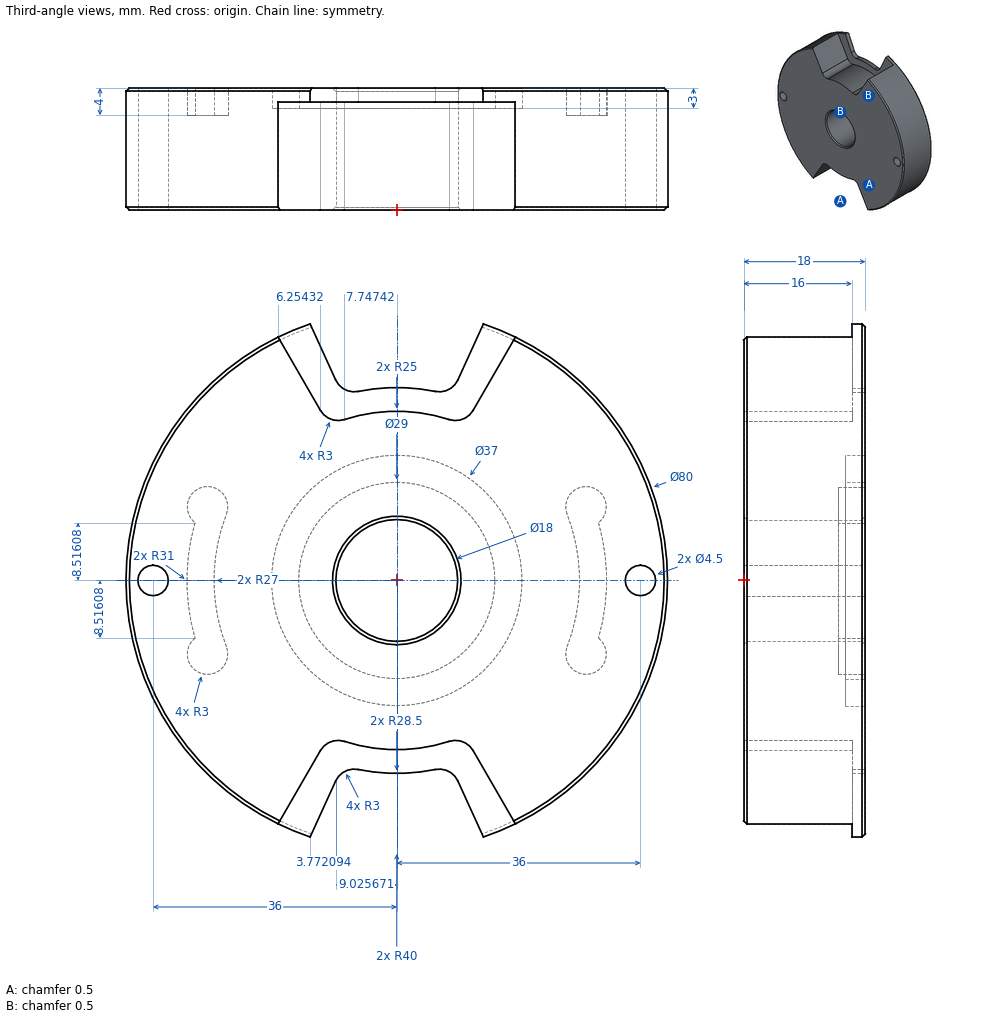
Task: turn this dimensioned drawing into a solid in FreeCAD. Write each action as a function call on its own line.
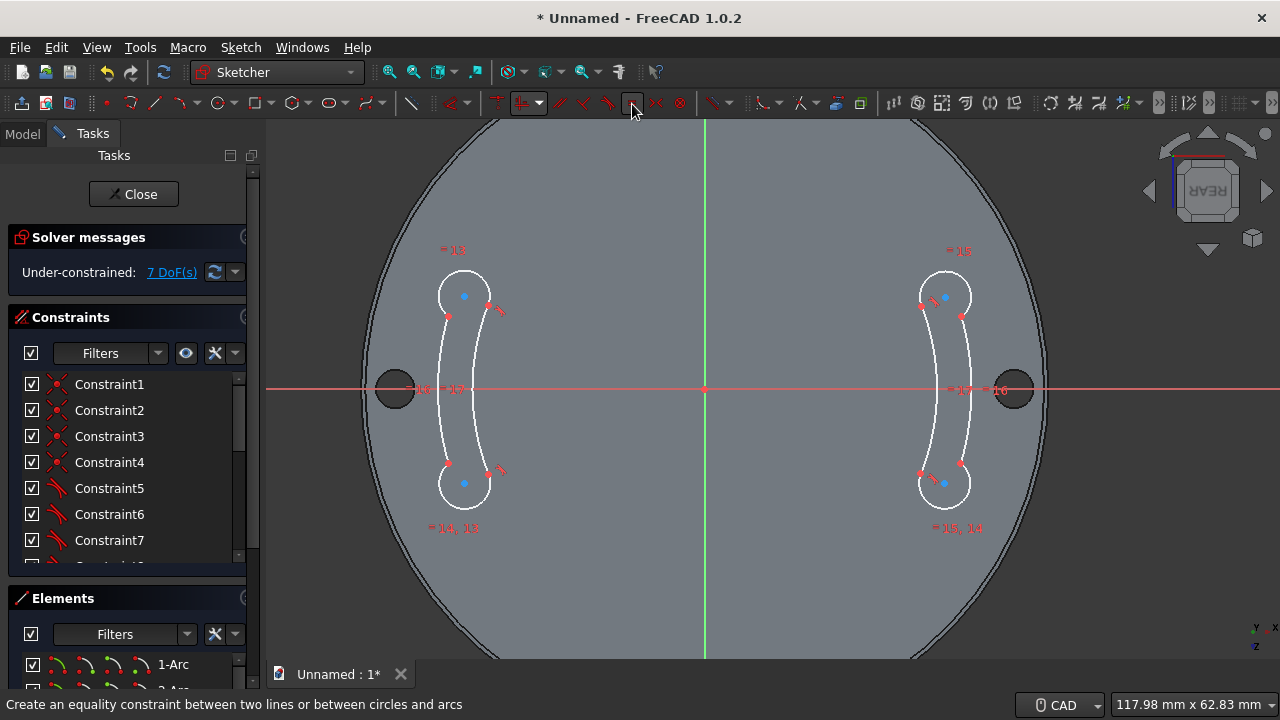
click(450, 104)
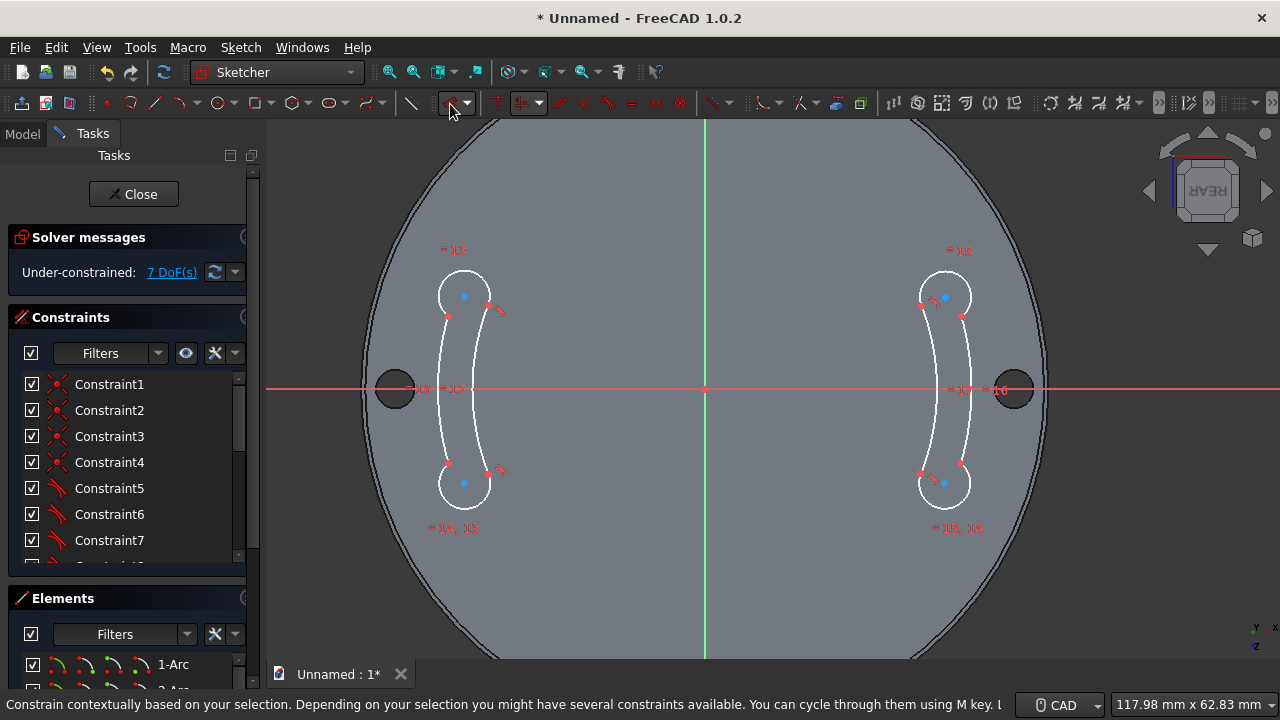
click(475, 355)
click(494, 230)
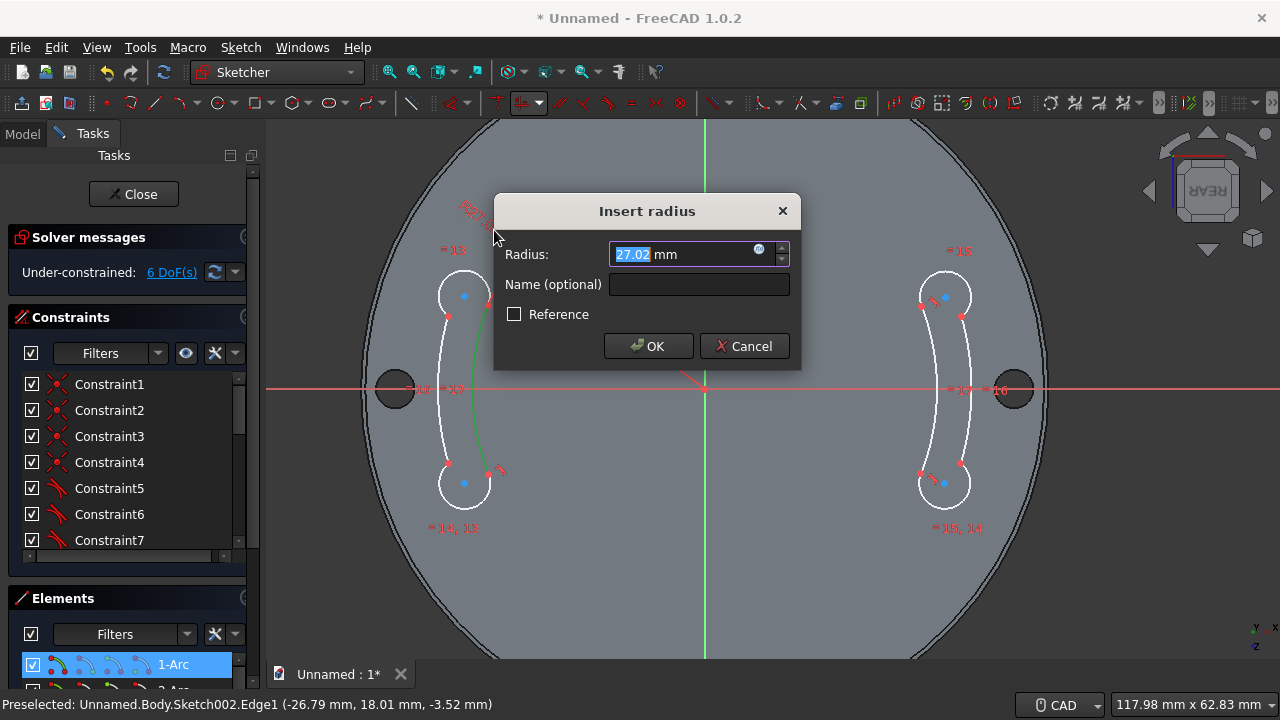
text(27)
key(Return)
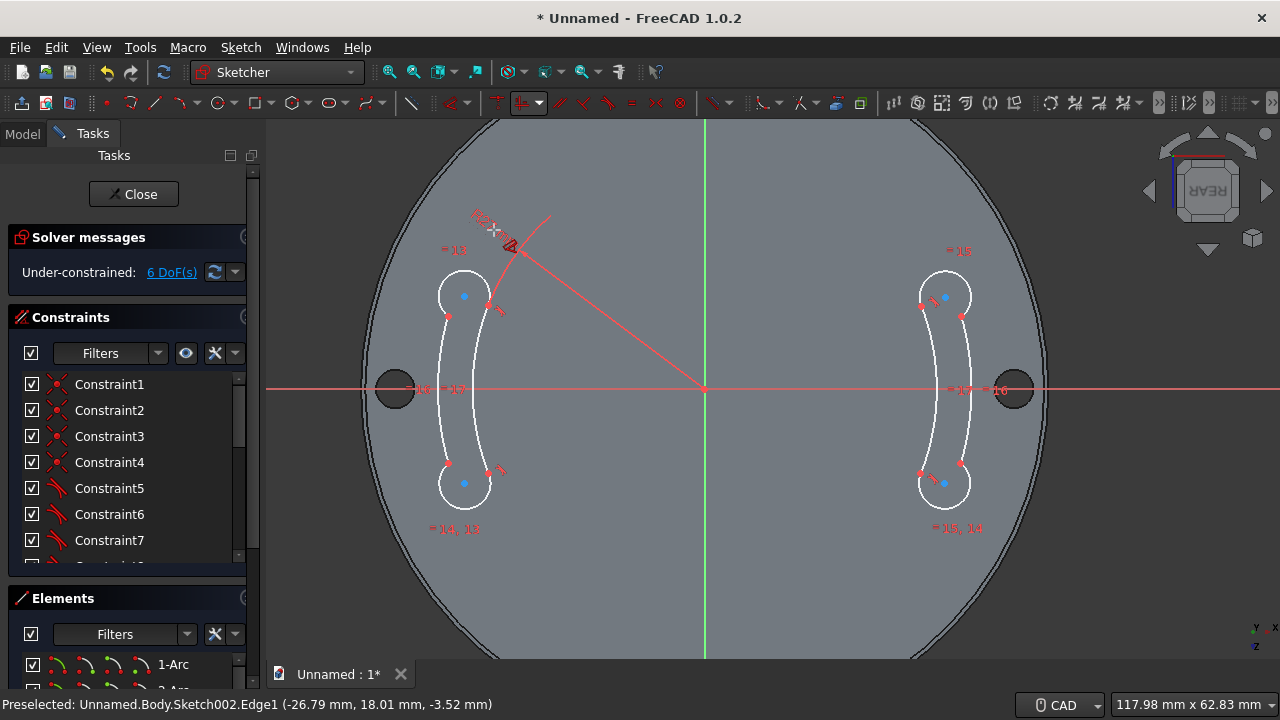
scroll(479, 275, up, 3)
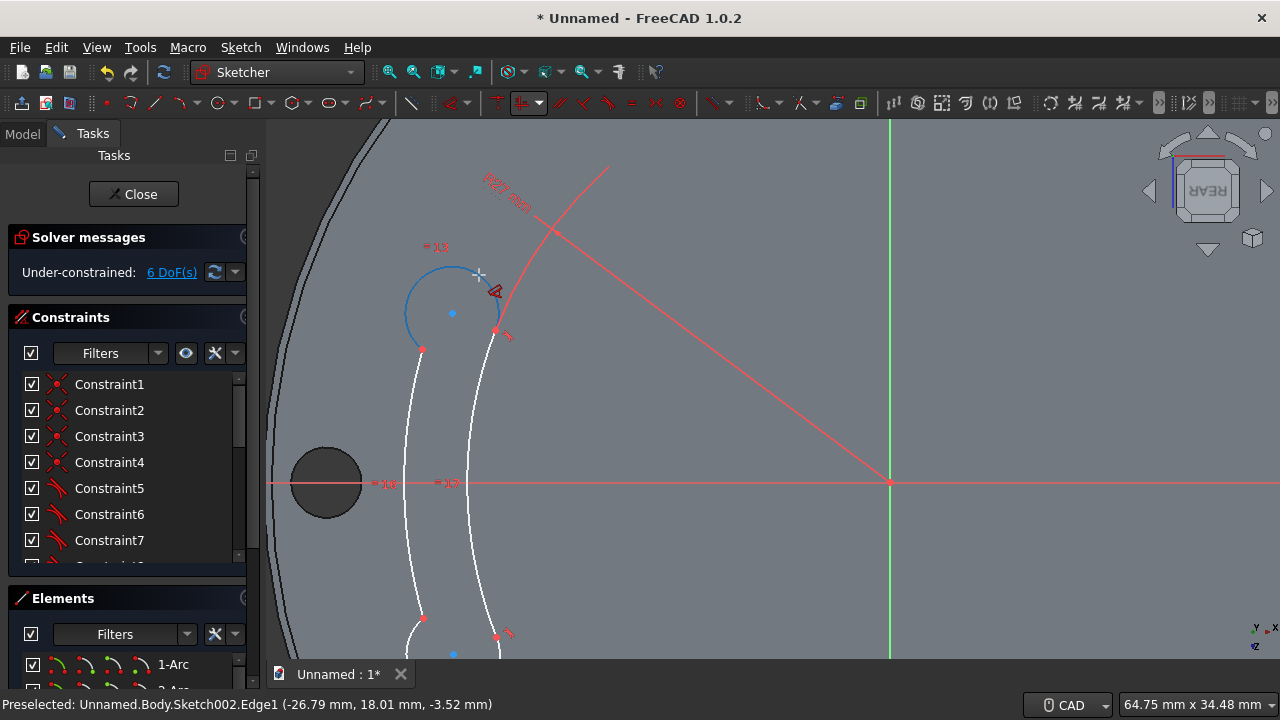
click(479, 275)
click(497, 249)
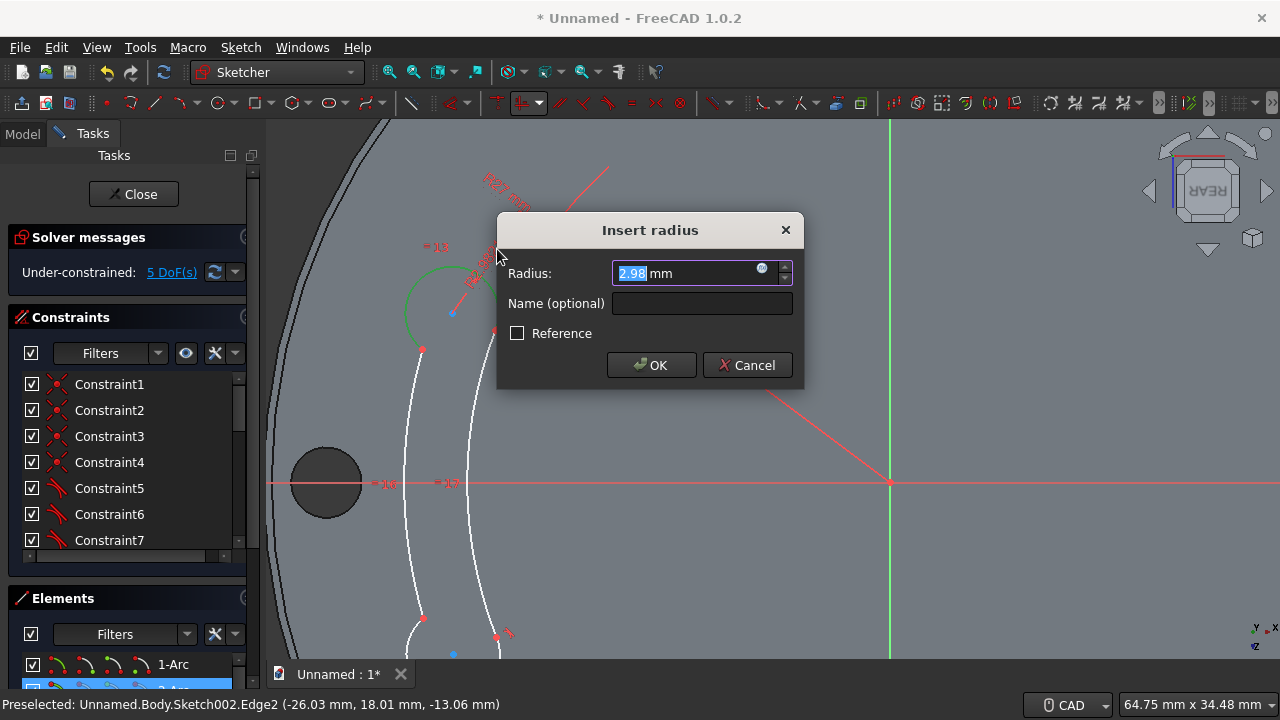
text(3)
key(Return)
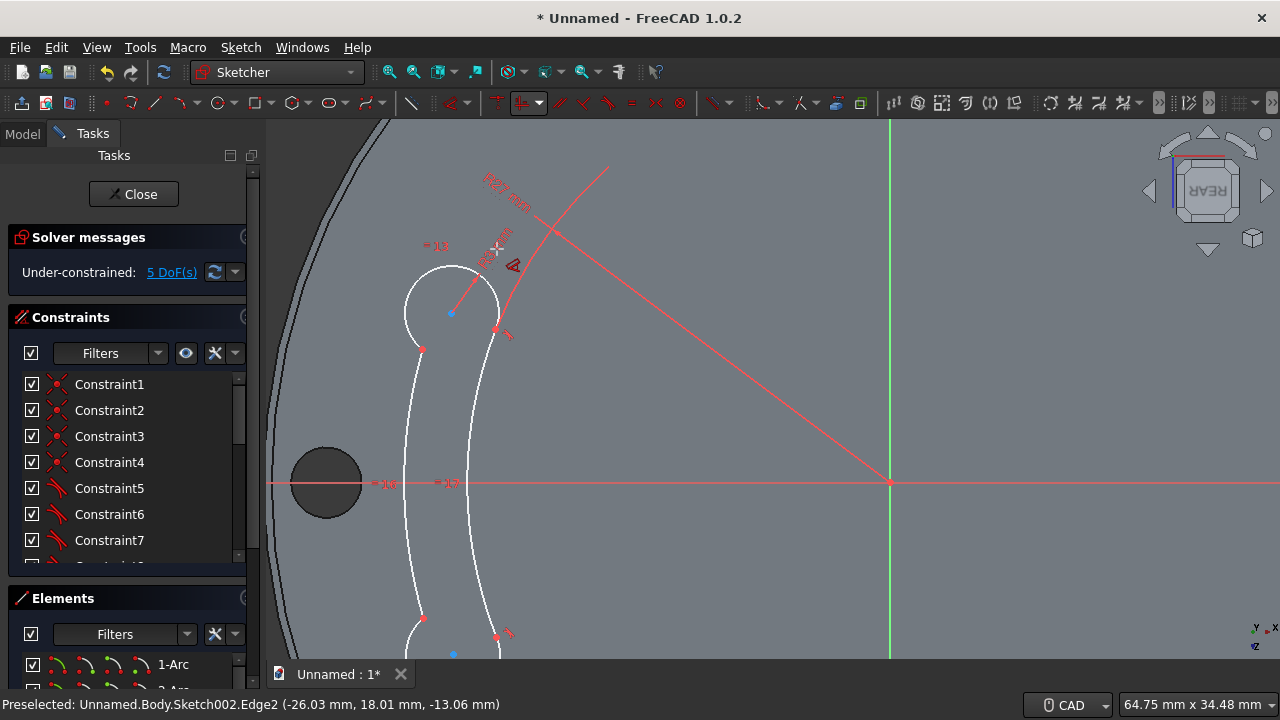
click(407, 430)
click(375, 427)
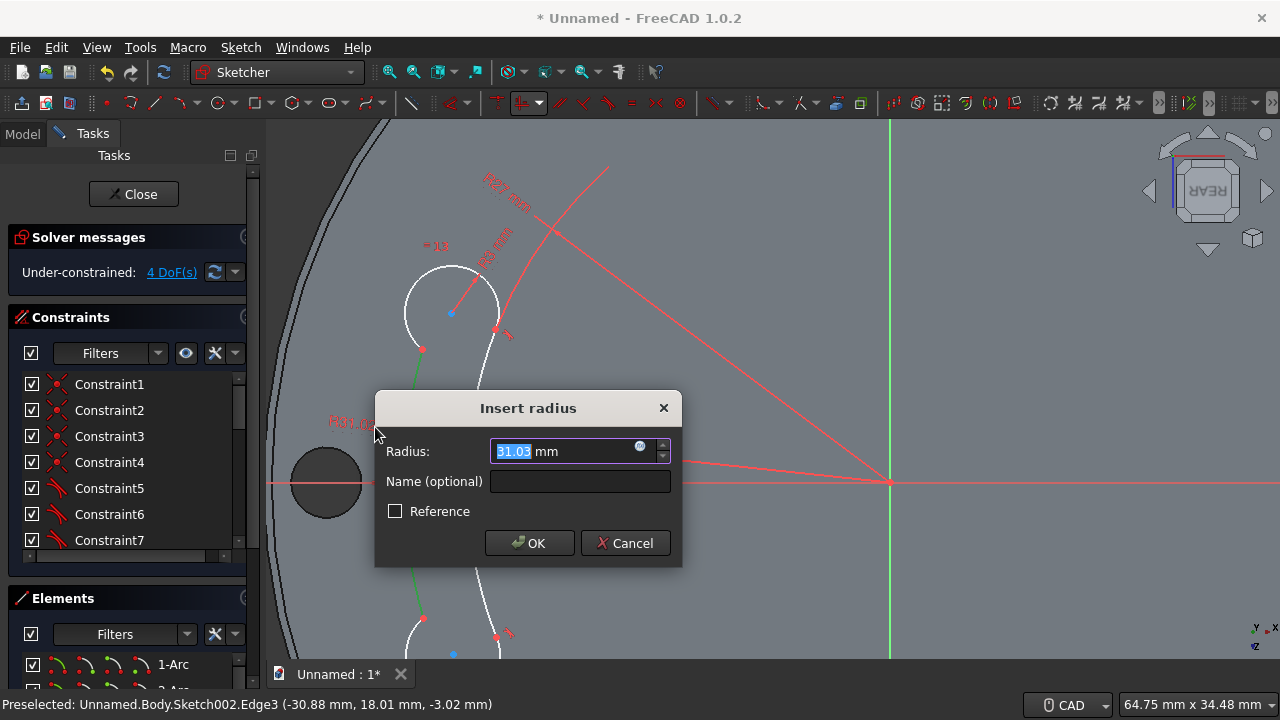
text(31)
key(Return)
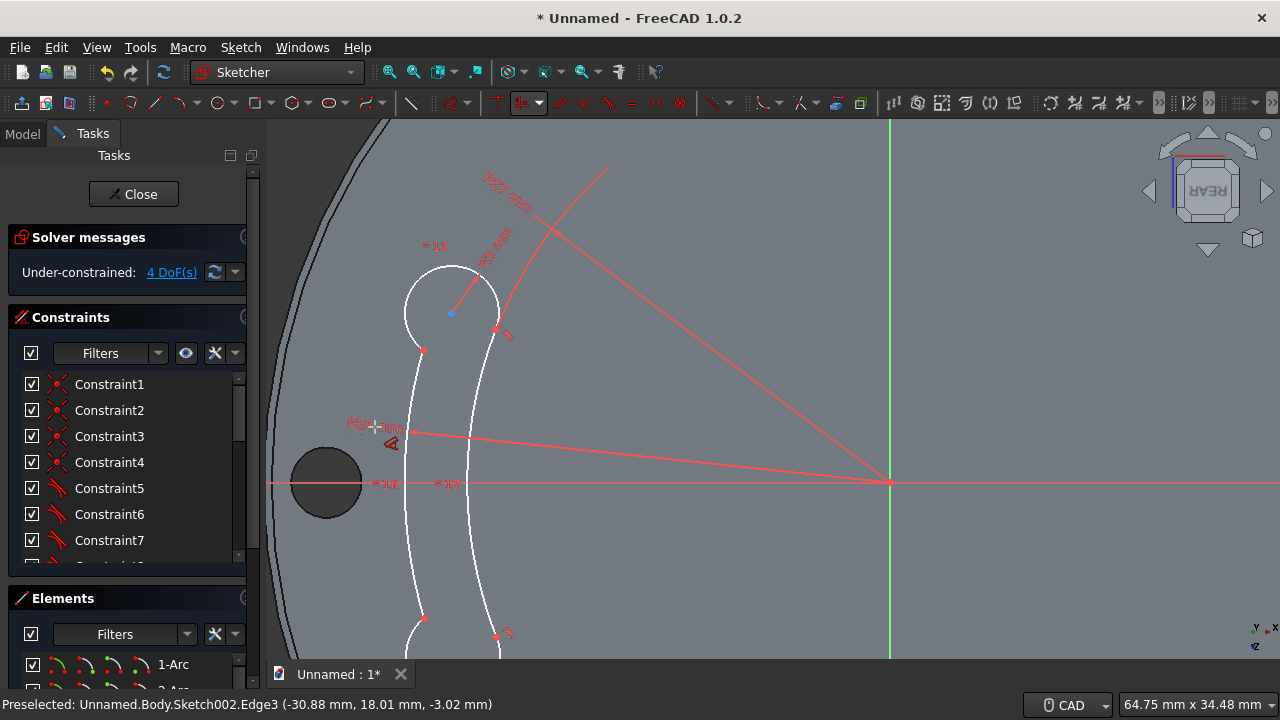
click(423, 350)
click(389, 386)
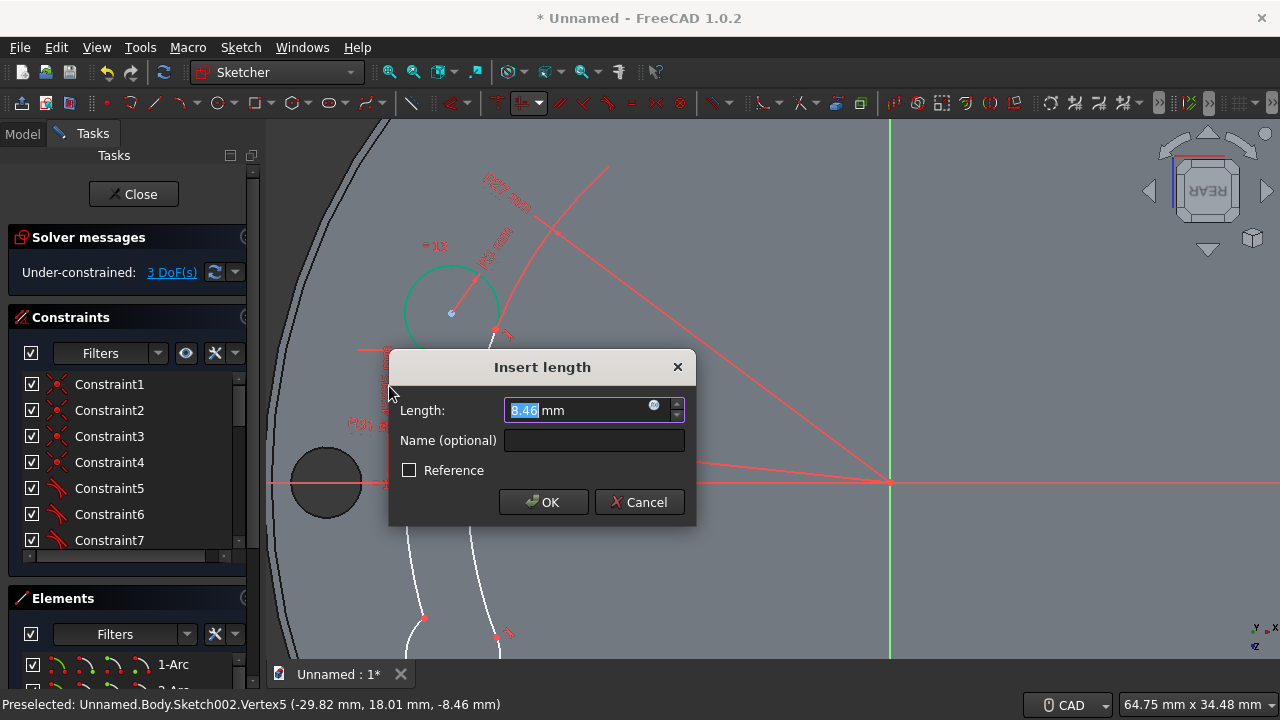
text(8.51608)
key(Return)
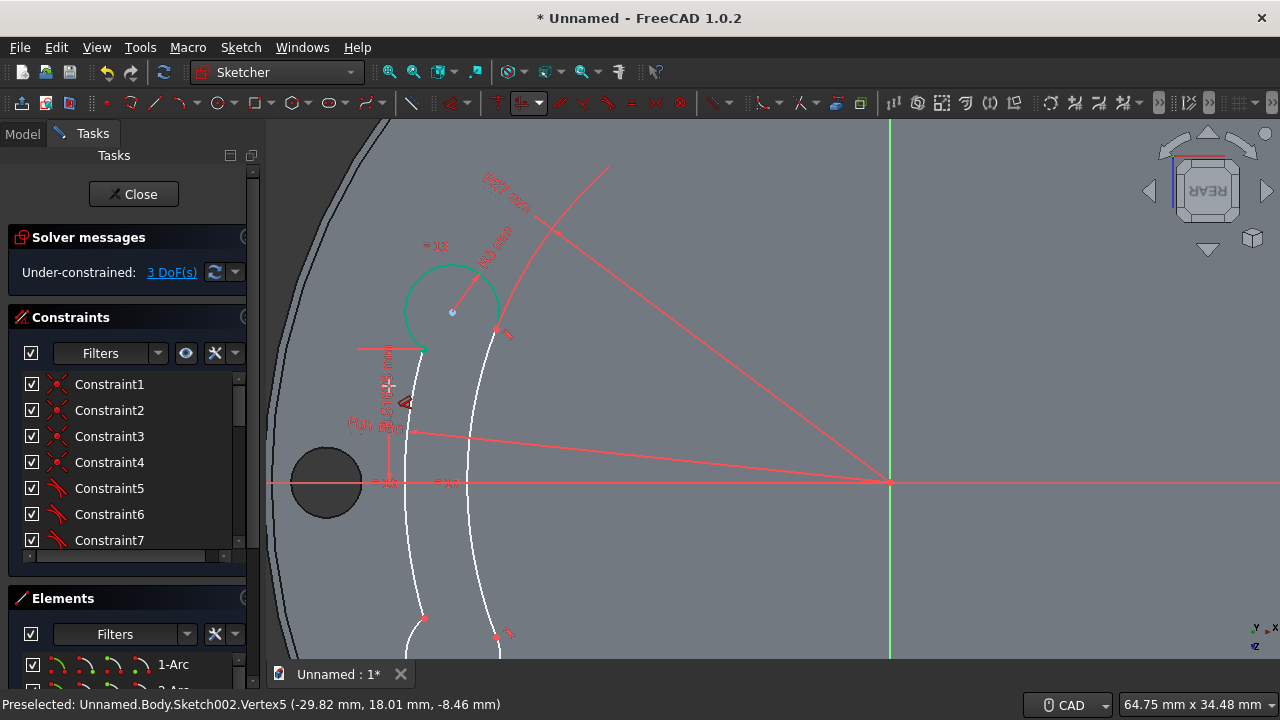
click(424, 618)
click(390, 550)